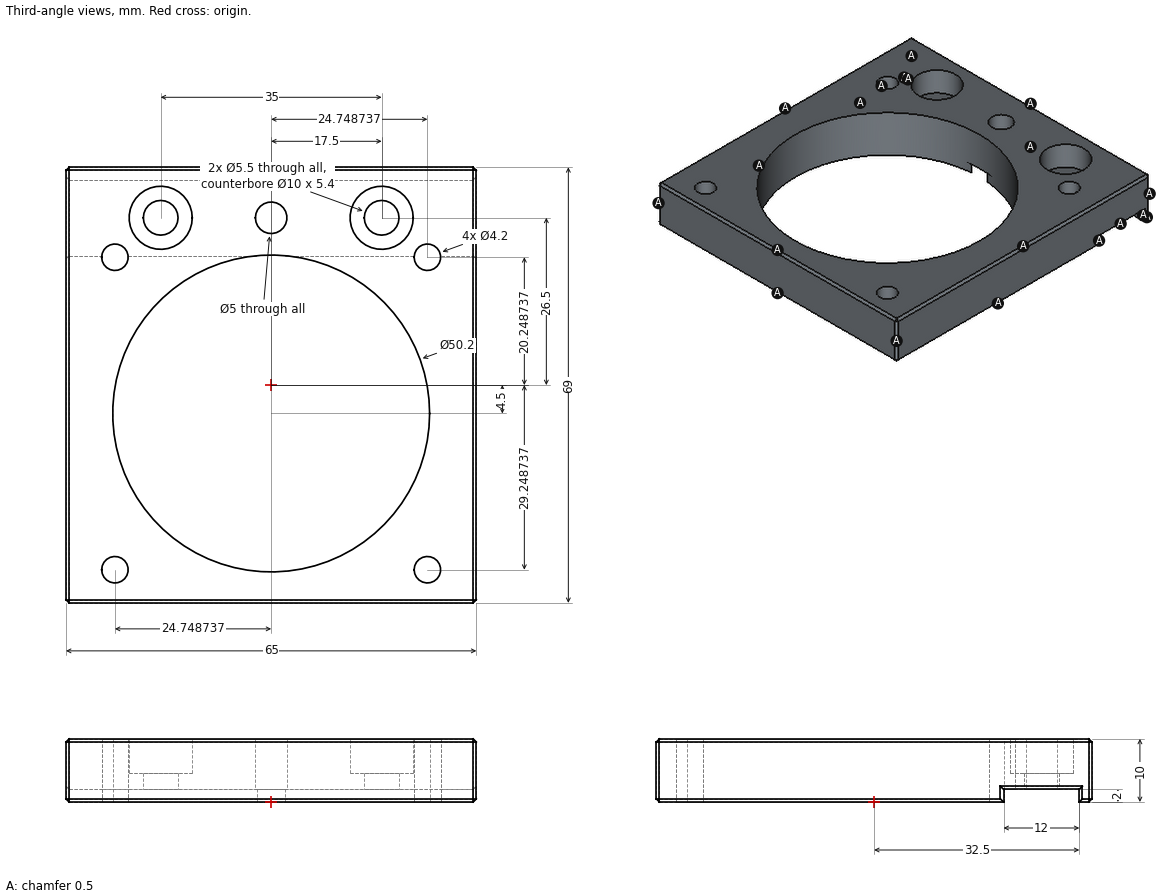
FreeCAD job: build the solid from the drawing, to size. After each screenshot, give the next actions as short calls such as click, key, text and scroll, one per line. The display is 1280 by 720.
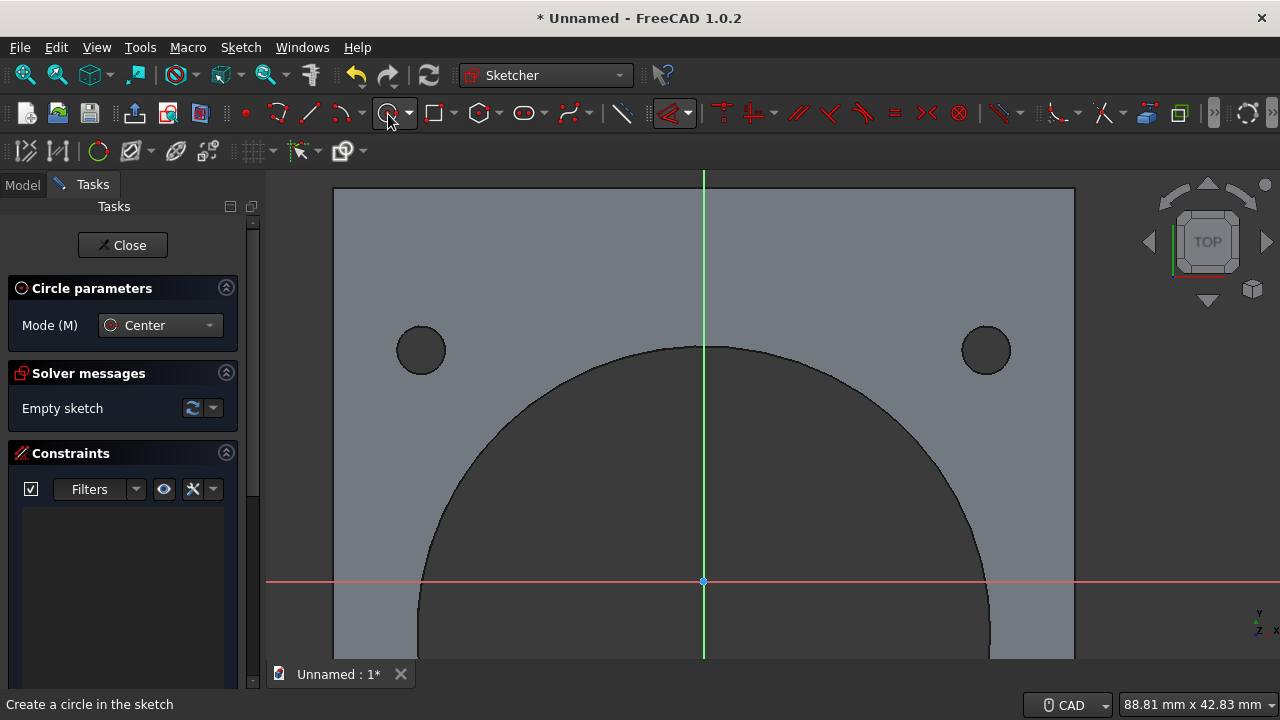
click(903, 279)
click(926, 257)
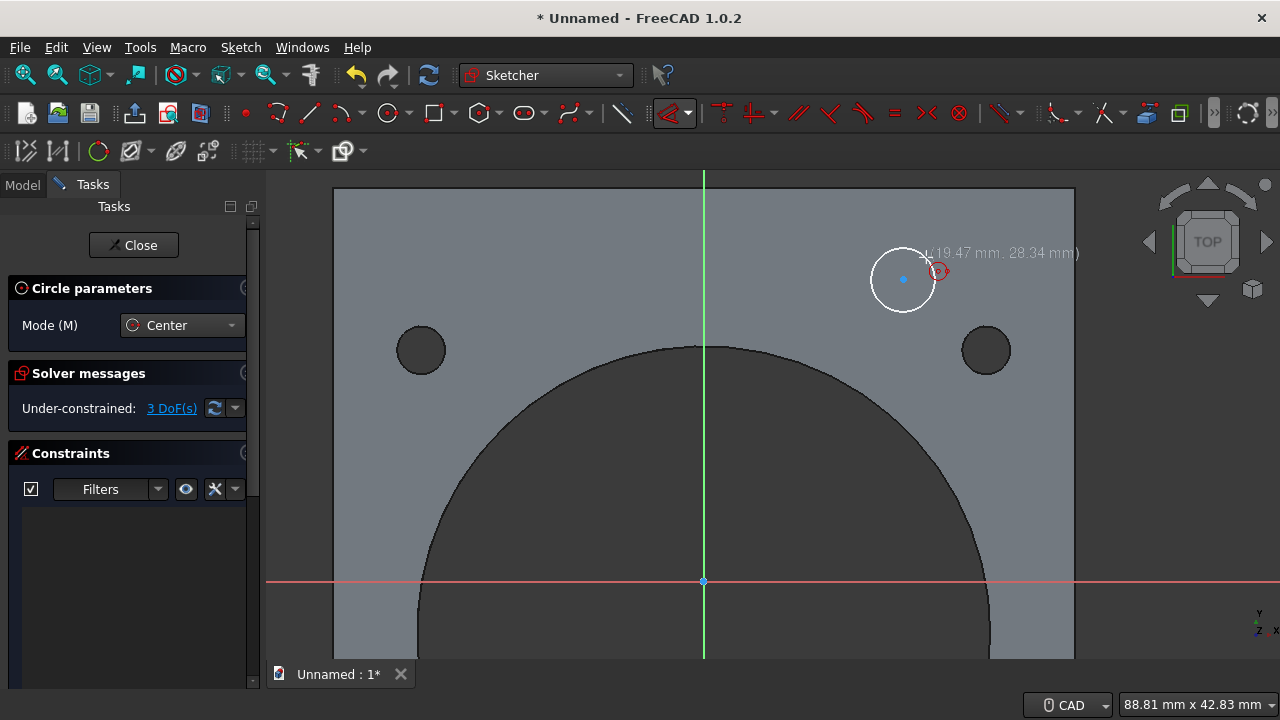
click(504, 279)
click(526, 257)
key(Escape)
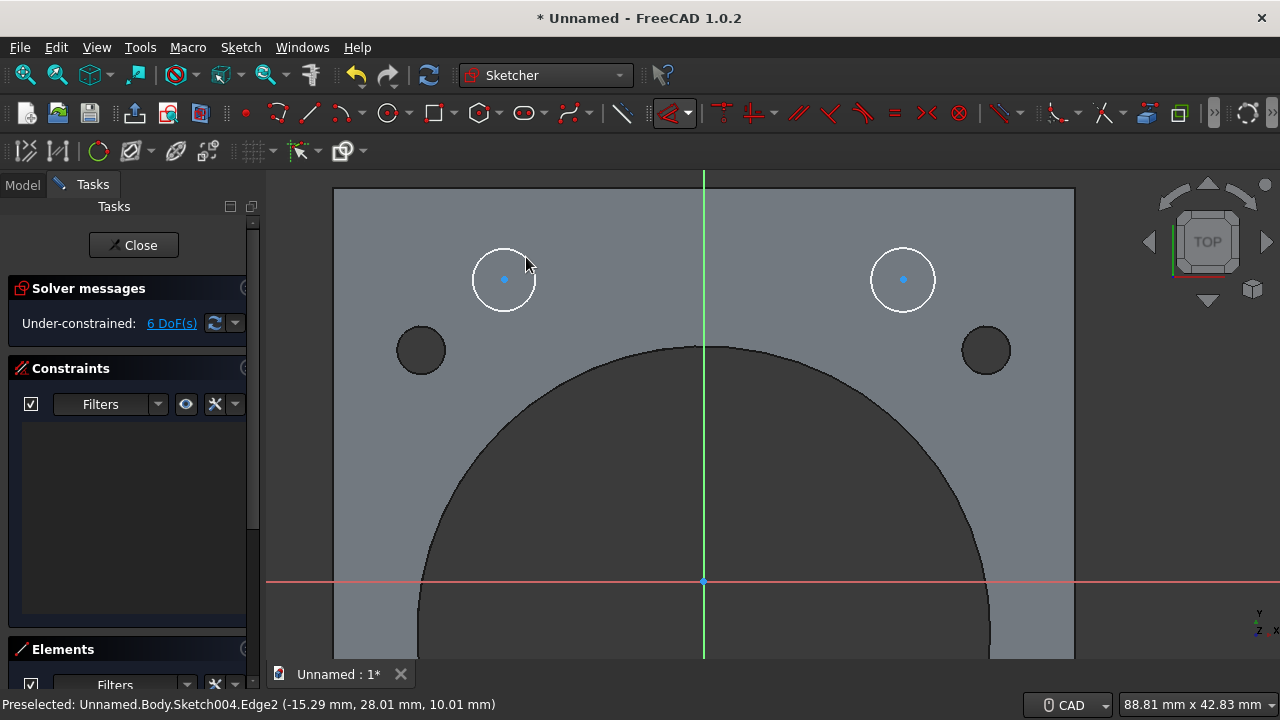
click(925, 257)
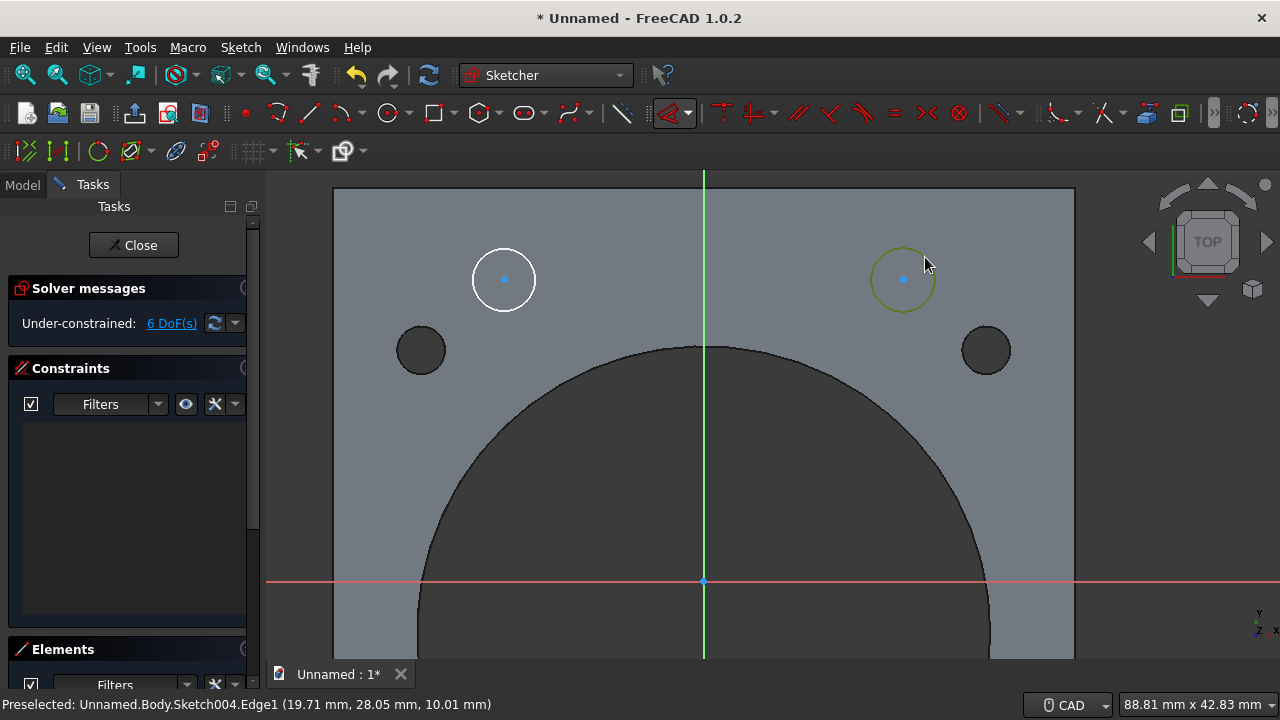
click(526, 258)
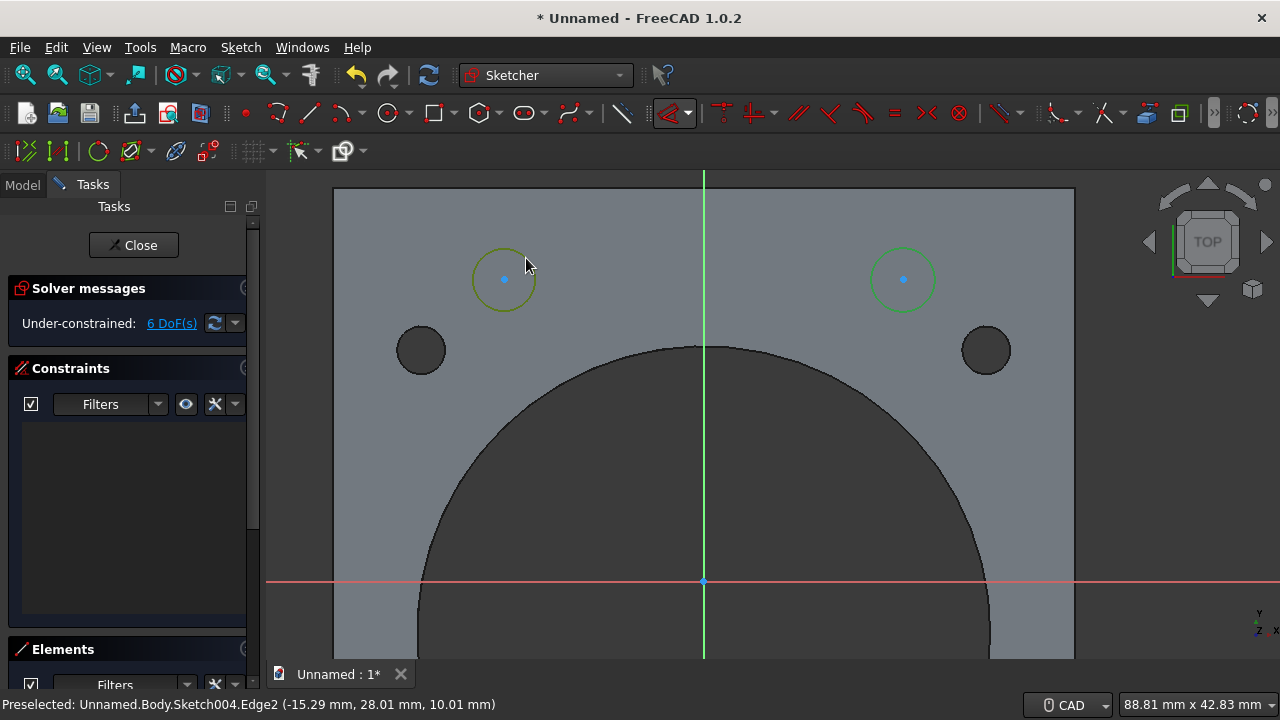
click(896, 114)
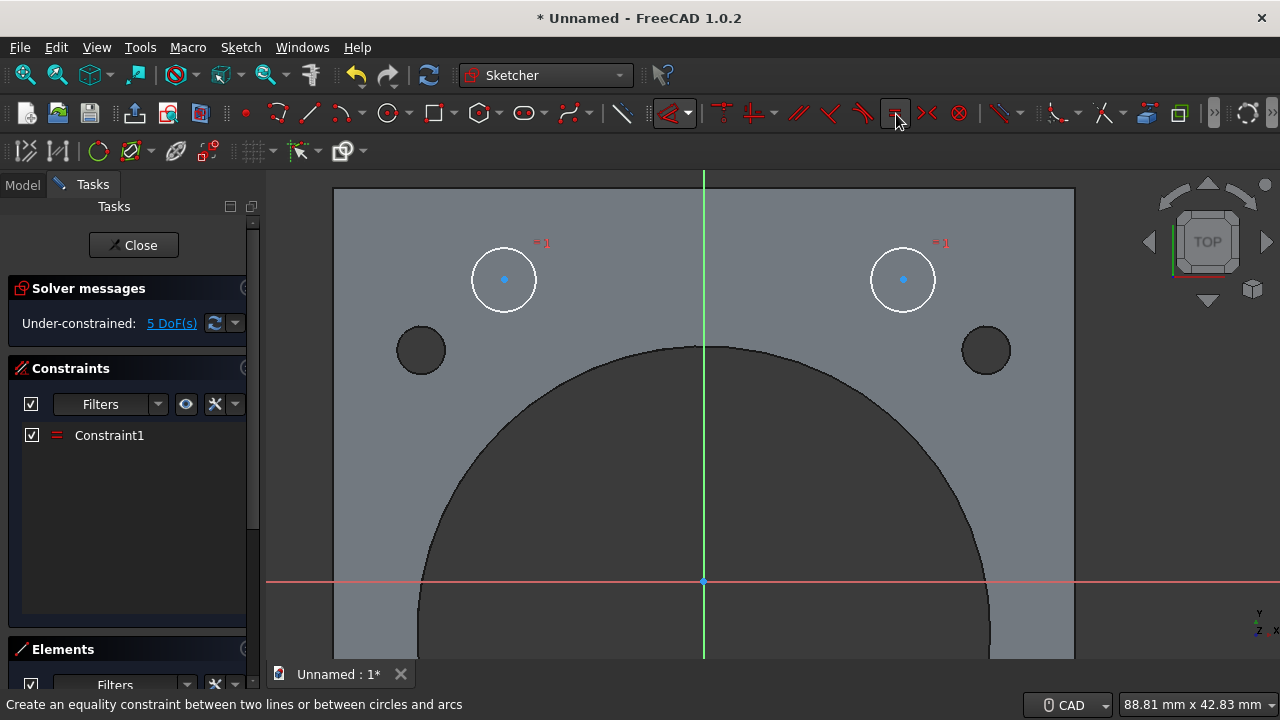
click(903, 280)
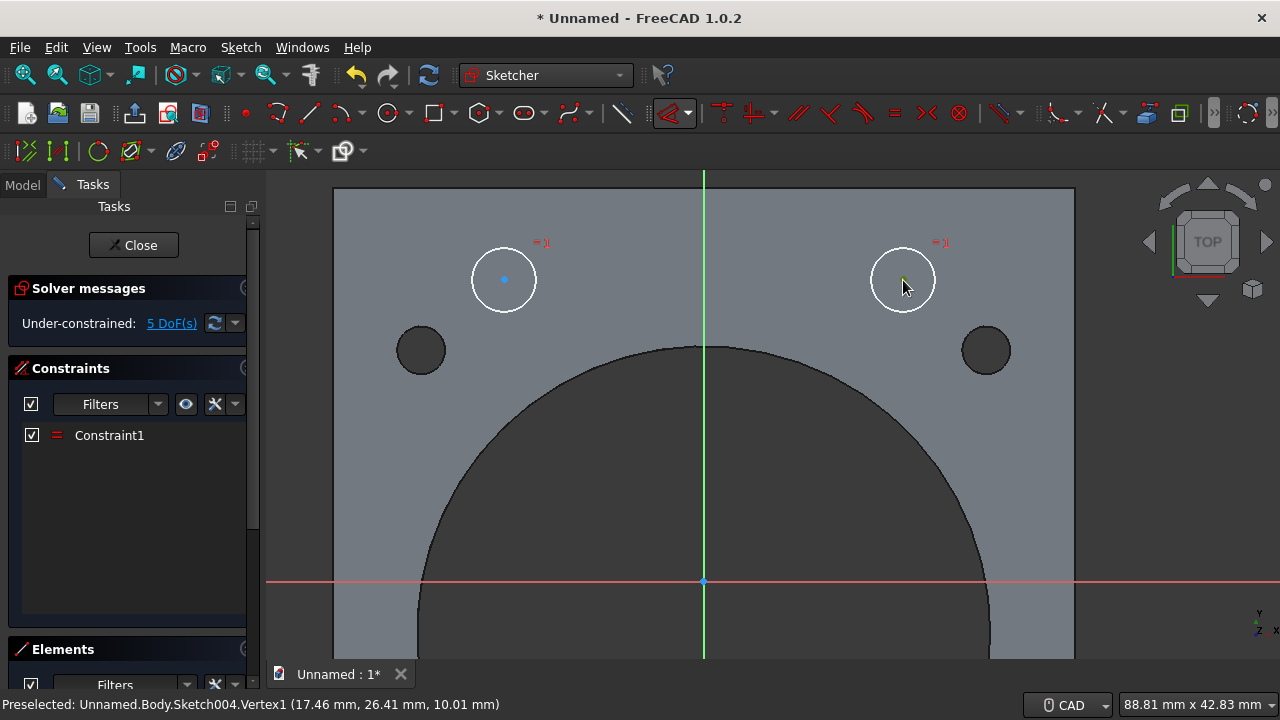
click(504, 280)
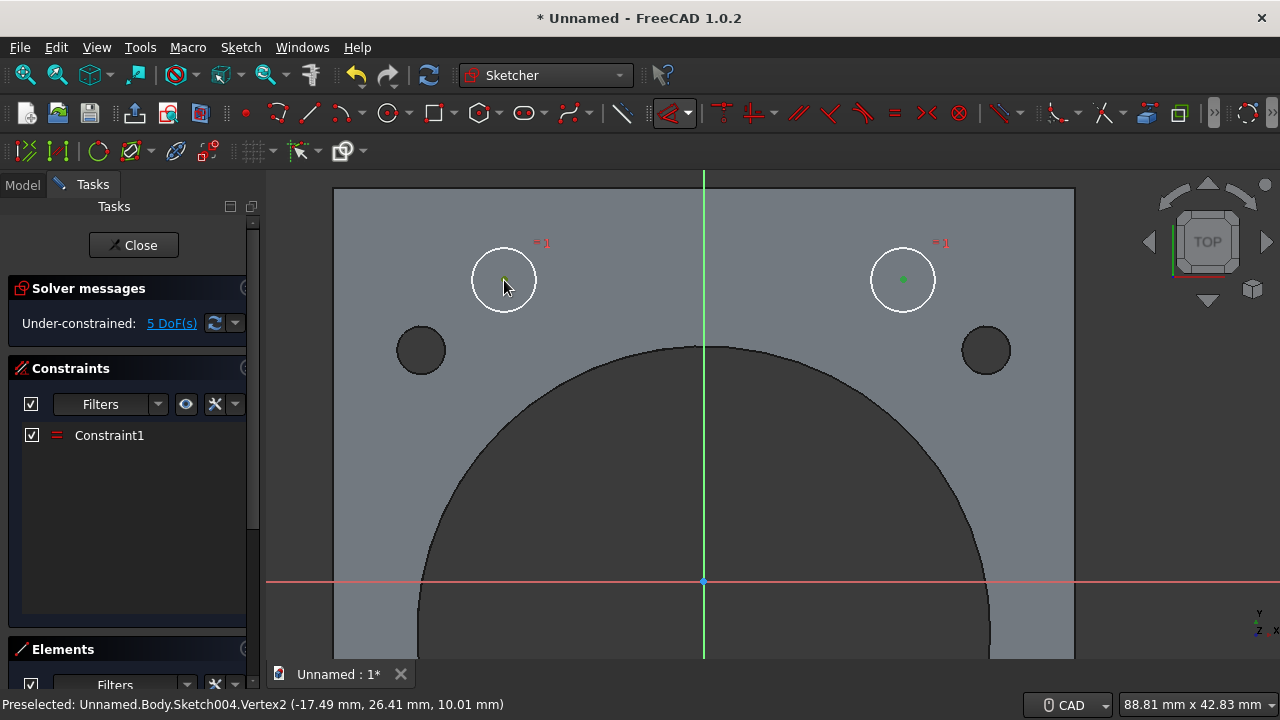
click(776, 114)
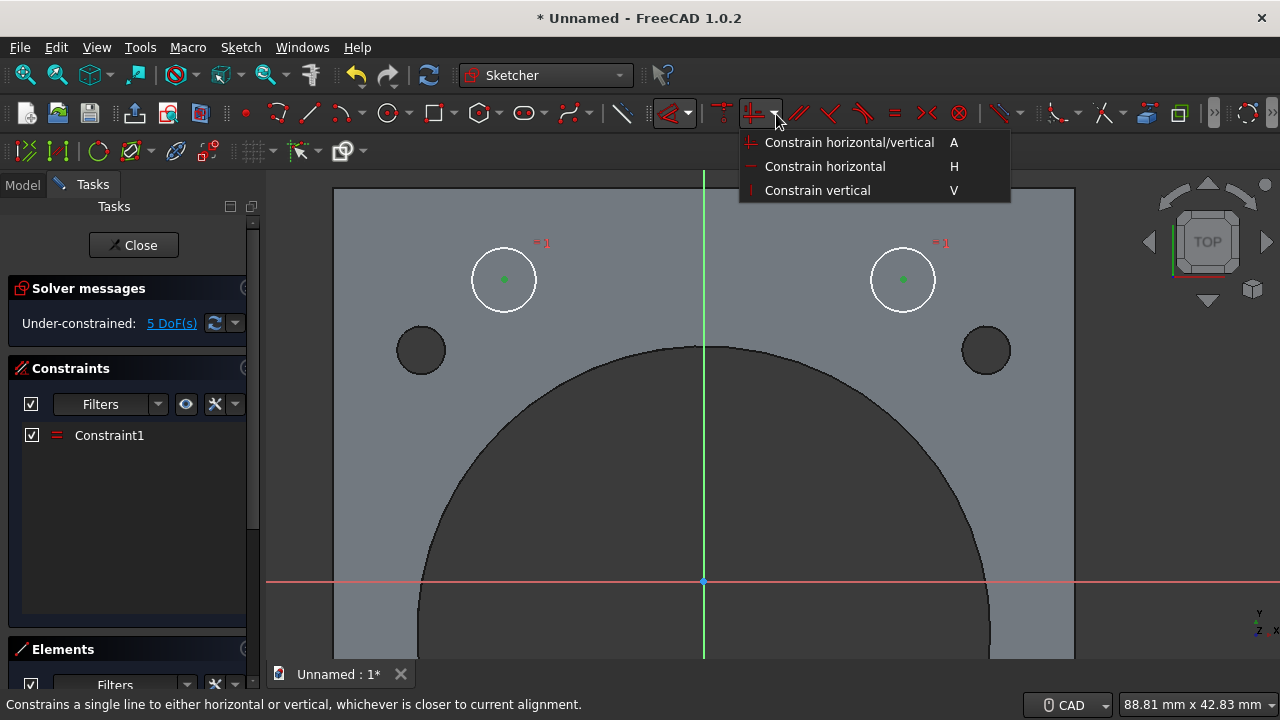
click(875, 166)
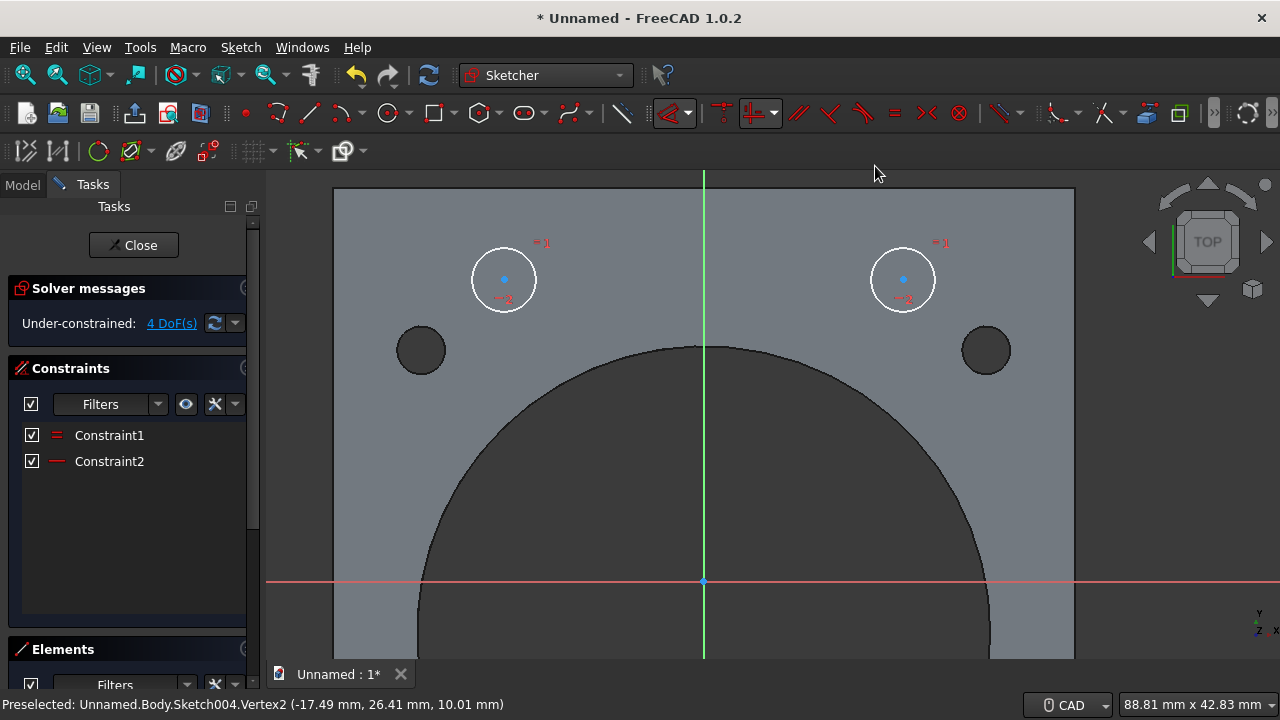
click(925, 257)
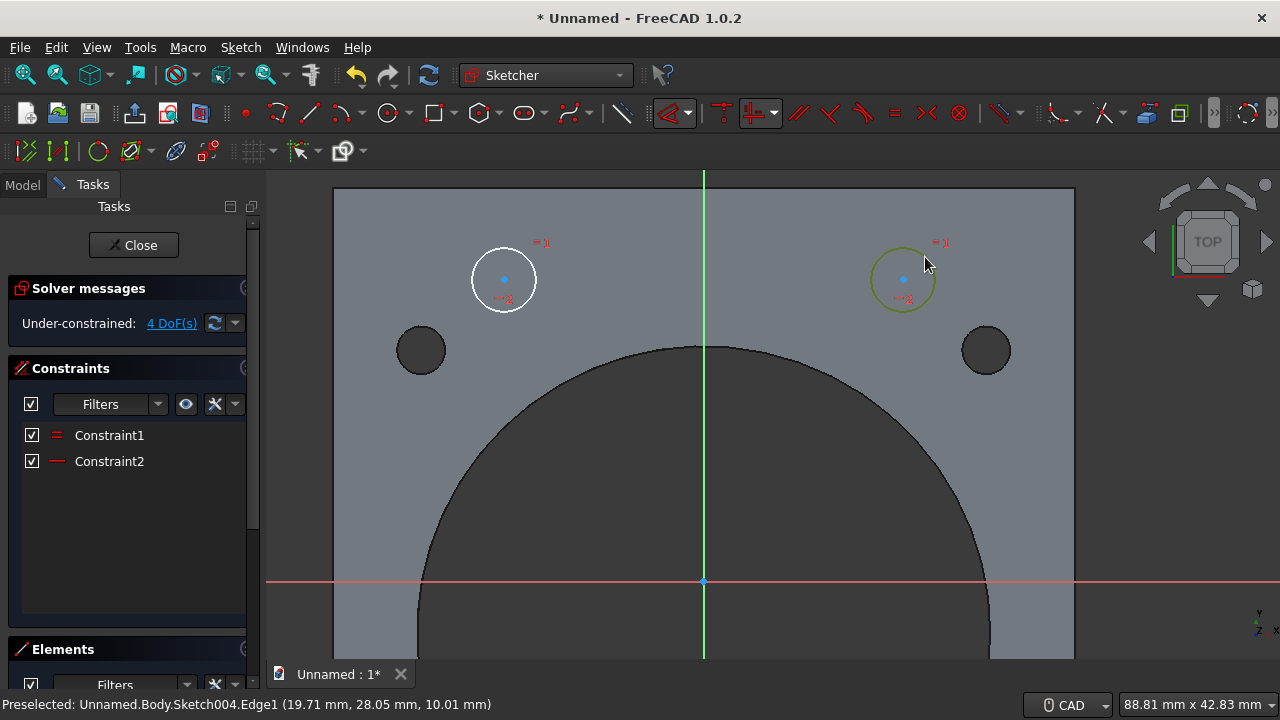
key(k)
key(o)